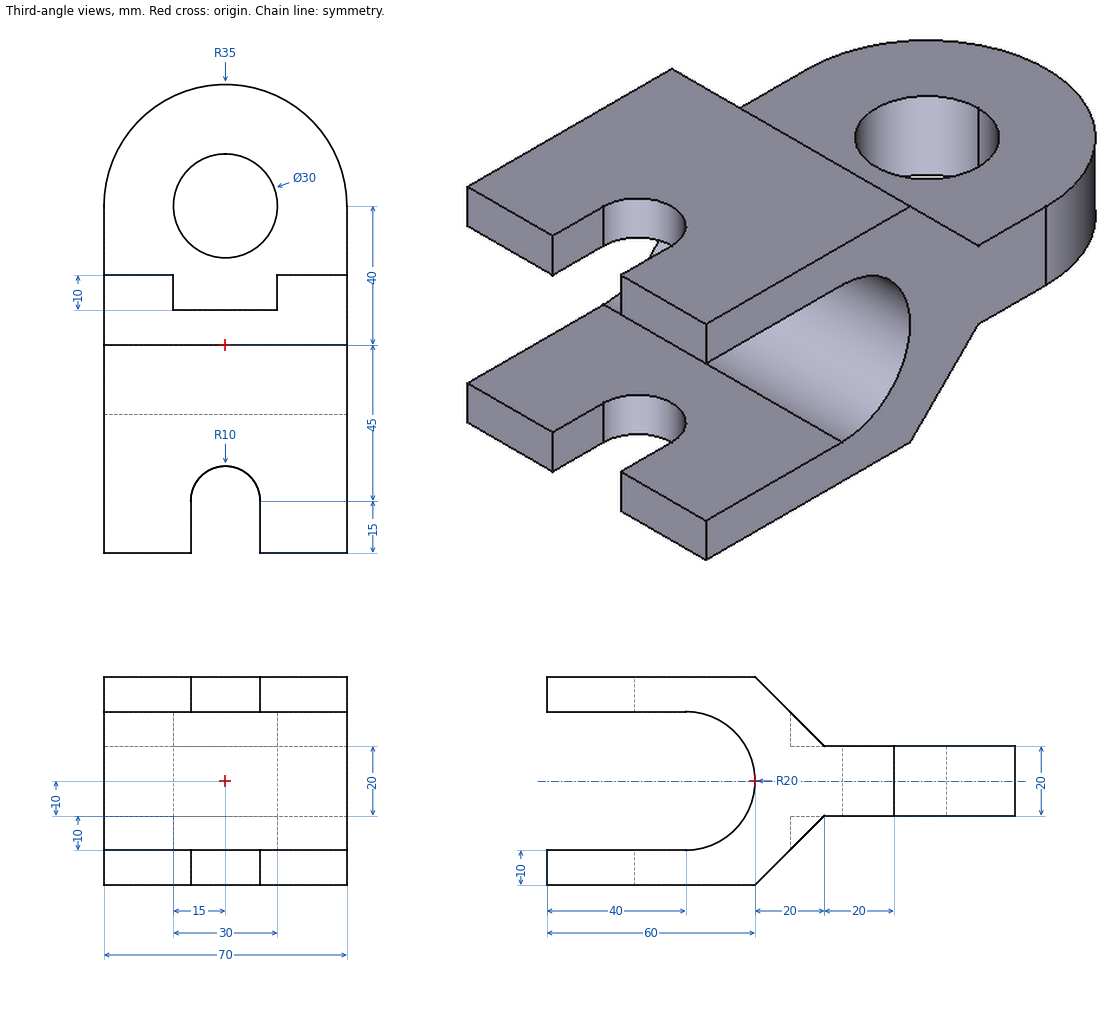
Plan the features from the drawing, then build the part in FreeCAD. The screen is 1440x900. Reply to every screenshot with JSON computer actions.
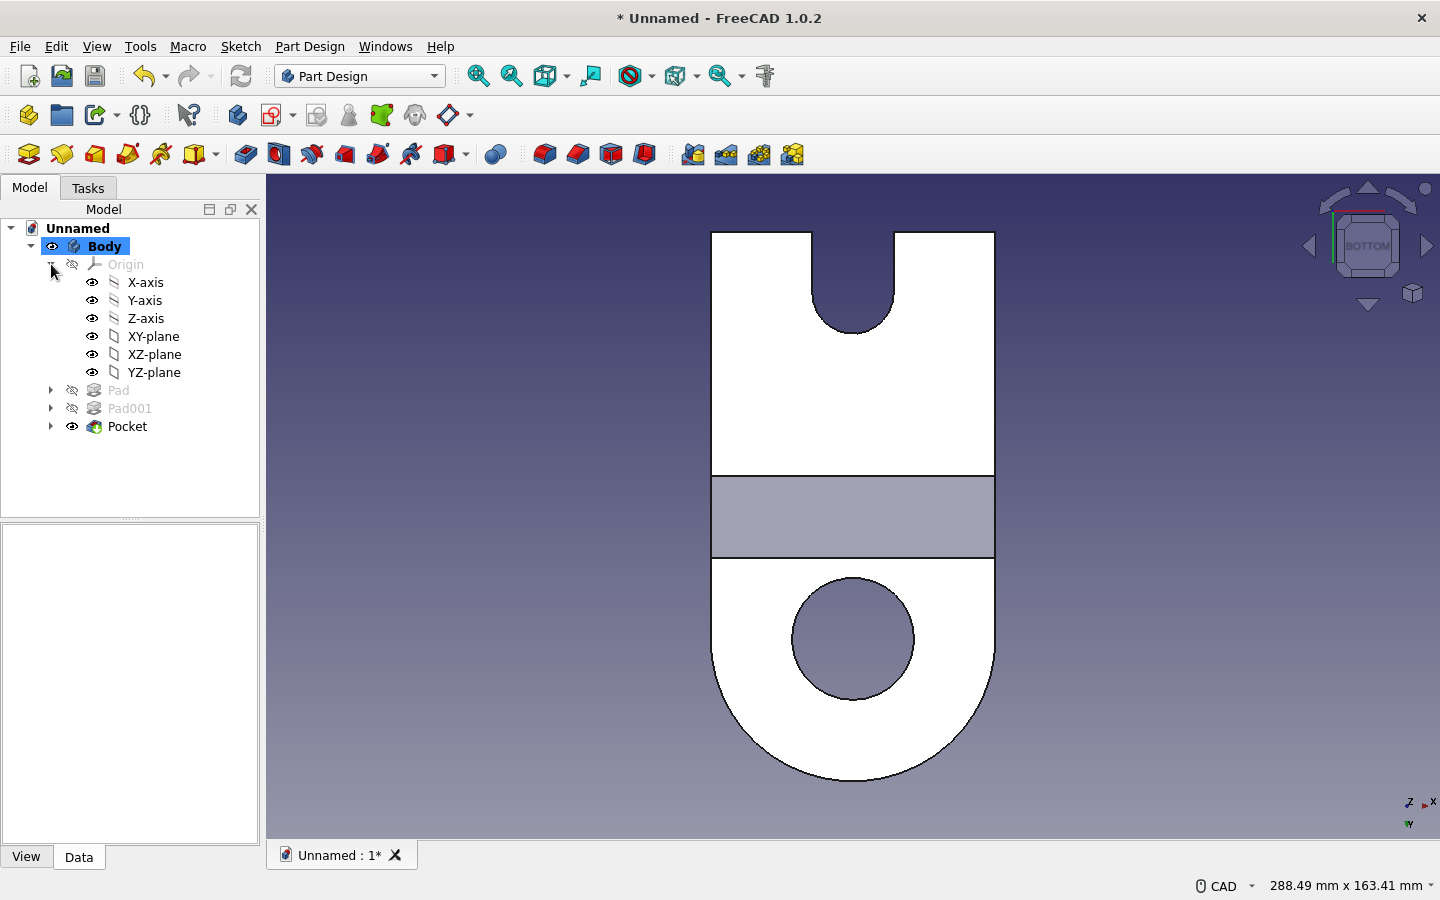
{"action": "left_click", "coordinate": [137, 354]}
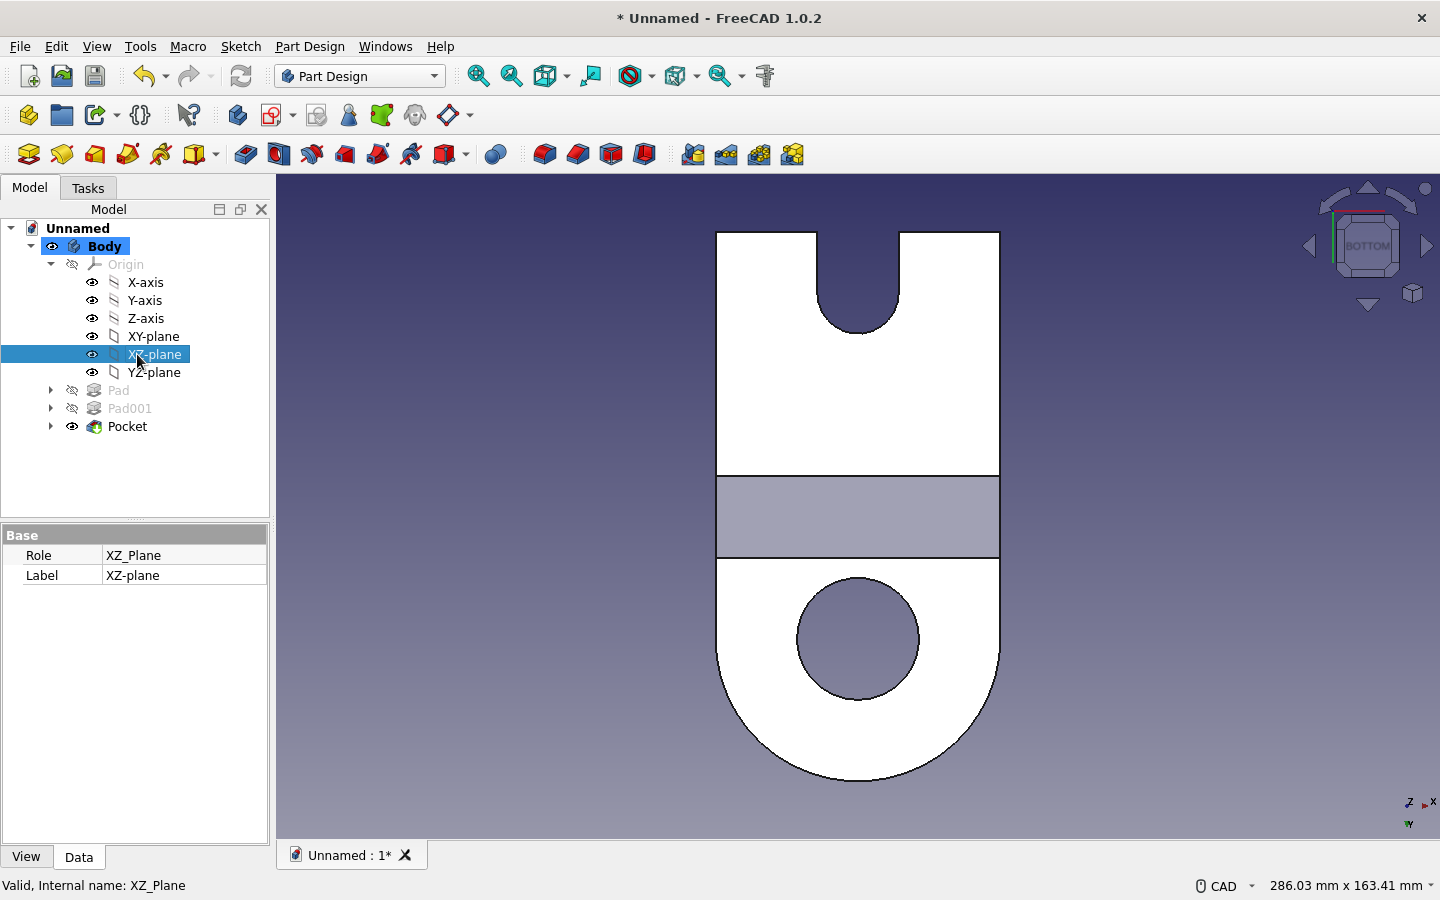
{"action": "left_click", "coordinate": [448, 116]}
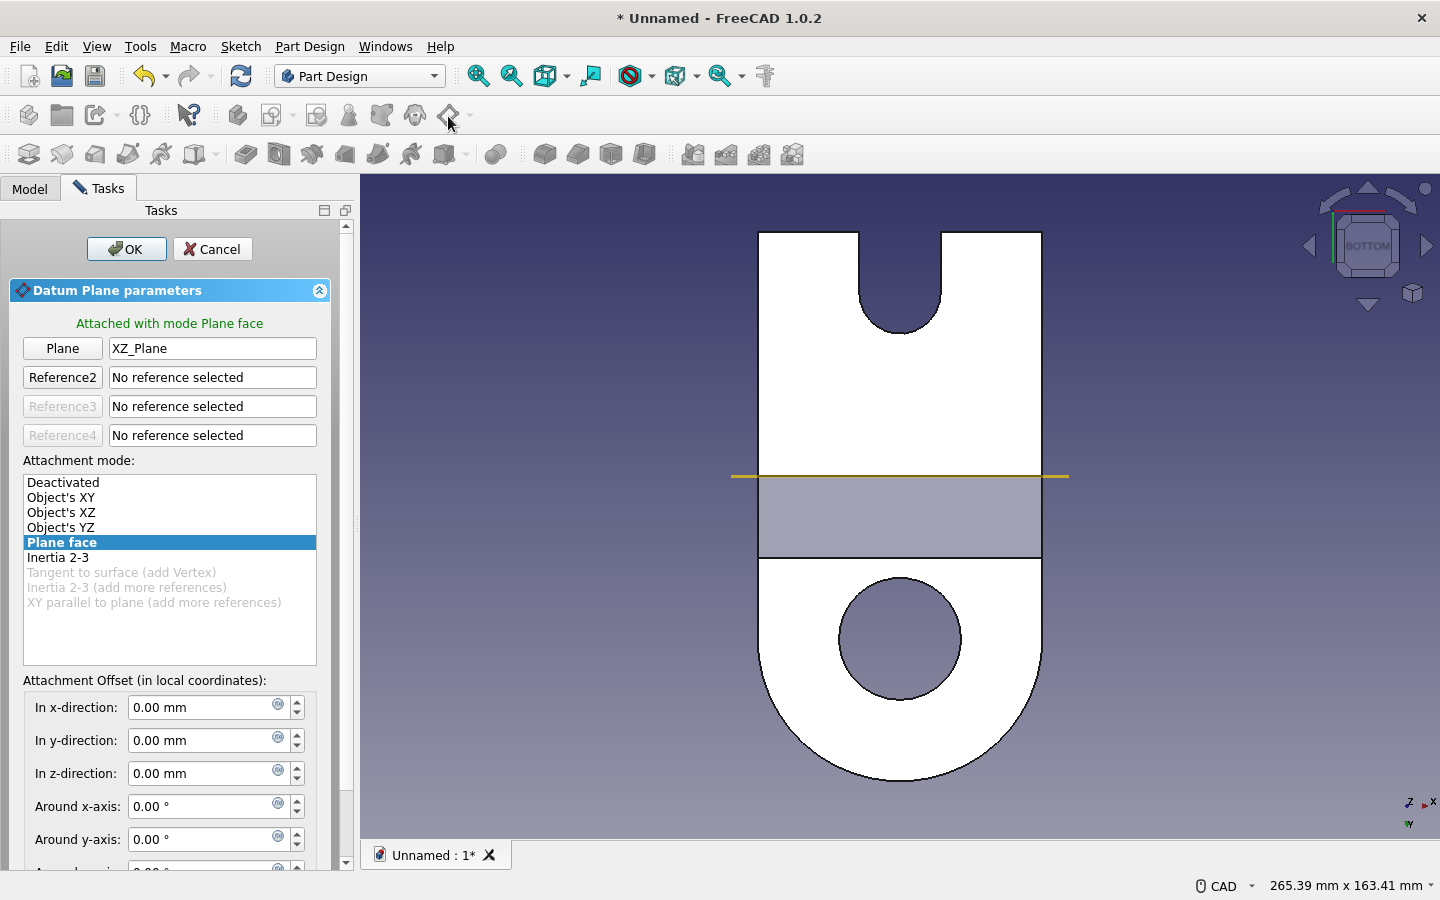
{"action": "triple_click", "coordinate": [210, 774]}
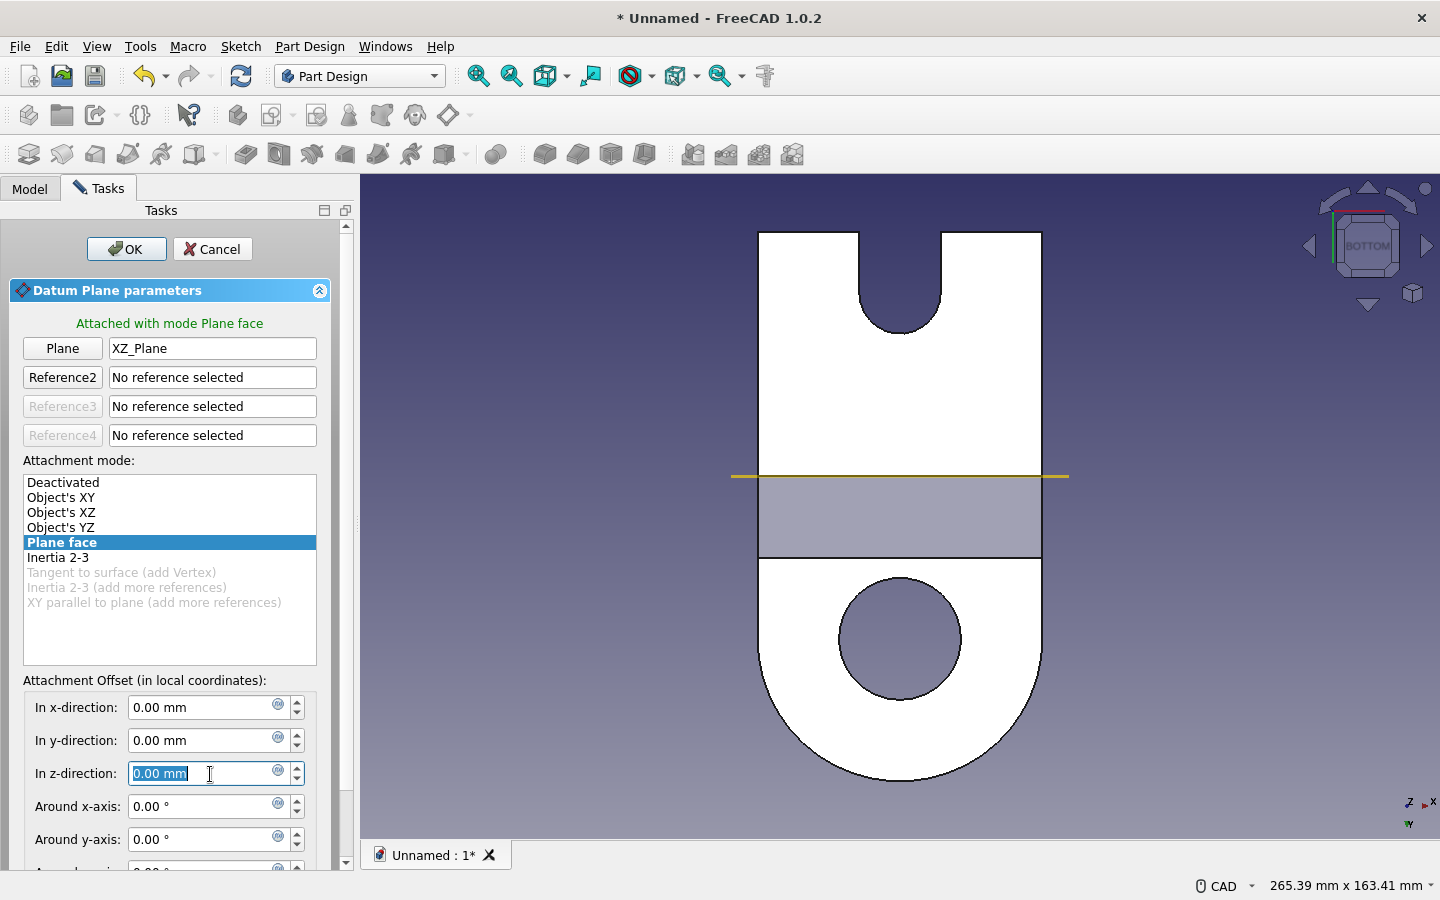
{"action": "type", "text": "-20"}
{"action": "key", "text": "Tab"}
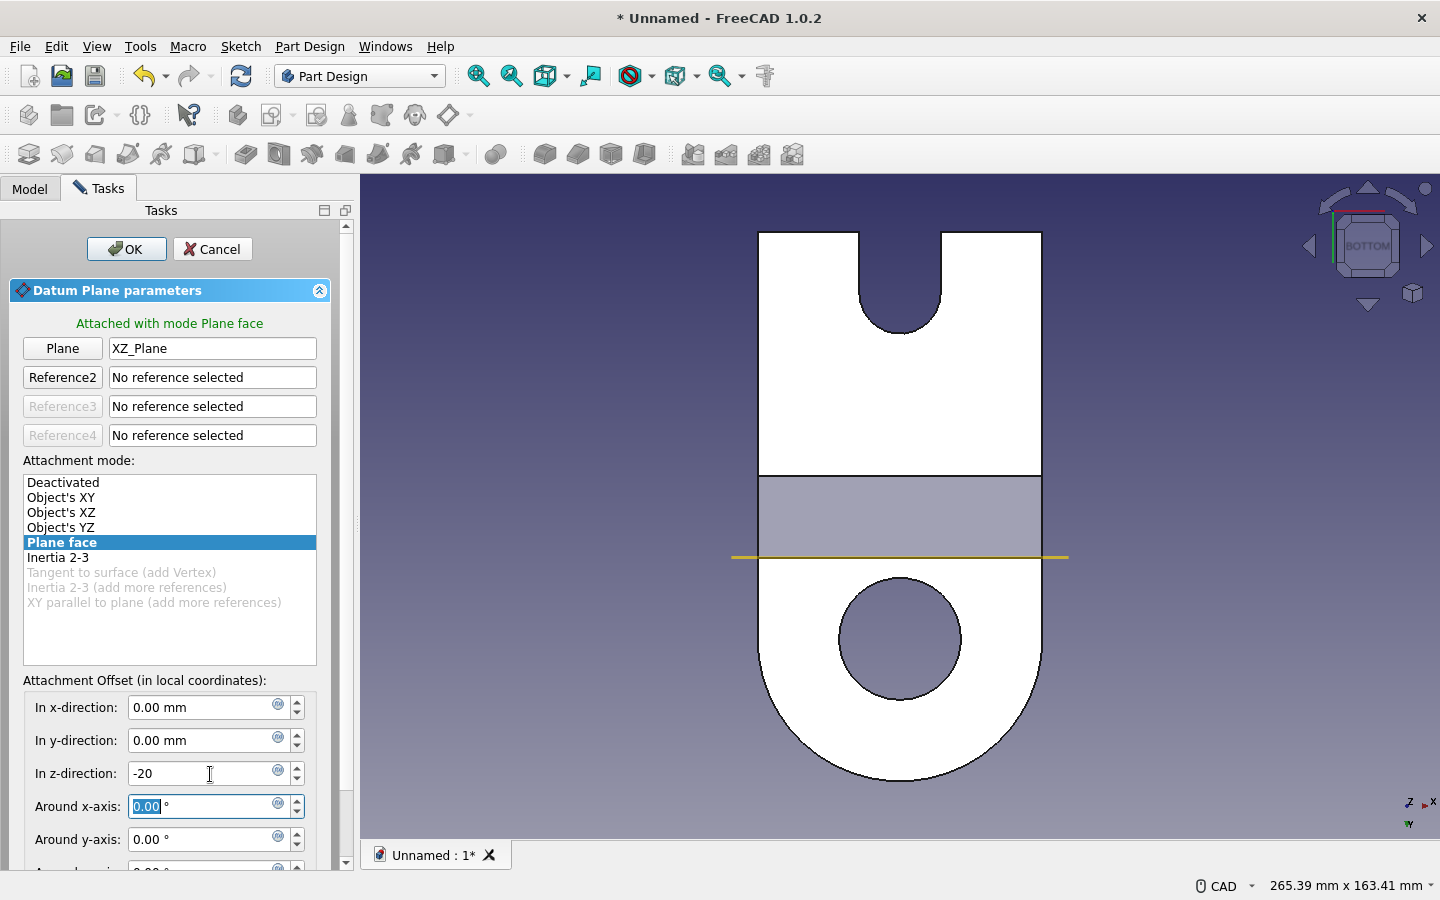
{"action": "left_click", "coordinate": [127, 249]}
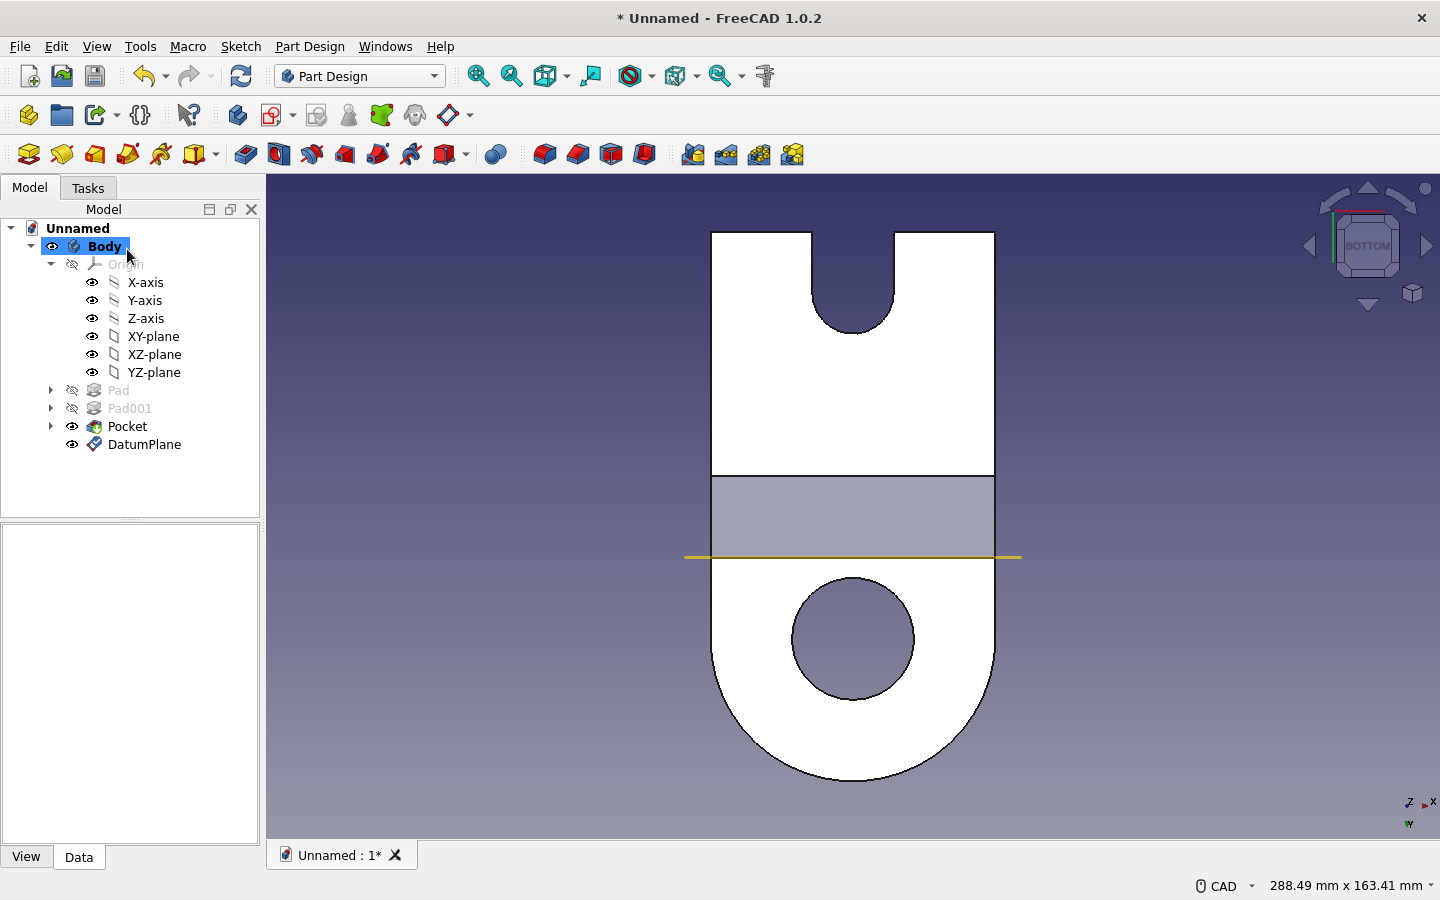
{"action": "left_click", "coordinate": [117, 444]}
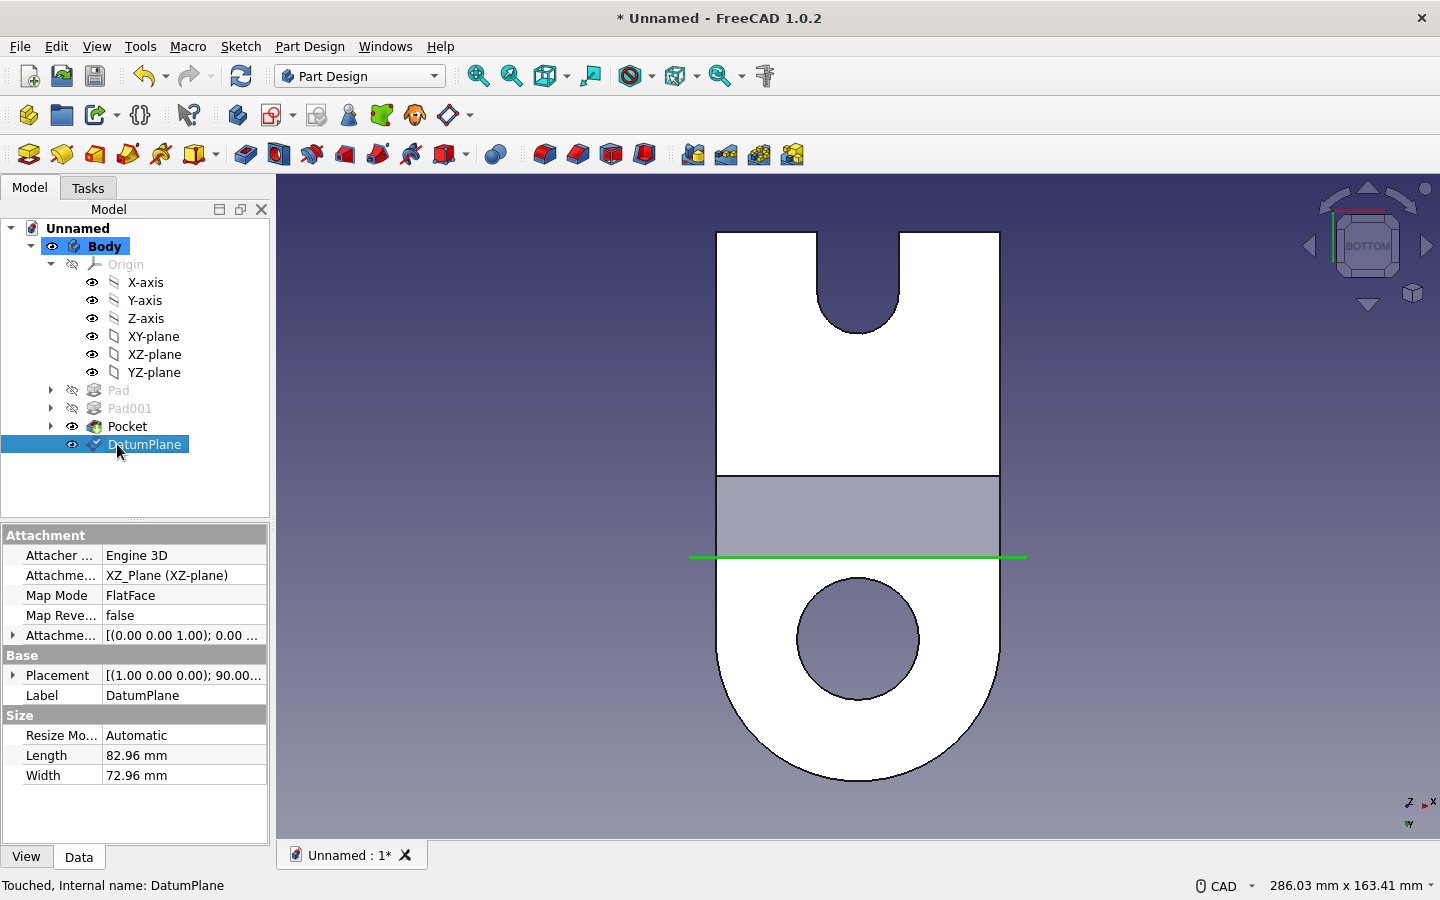
{"action": "left_click", "coordinate": [270, 116]}